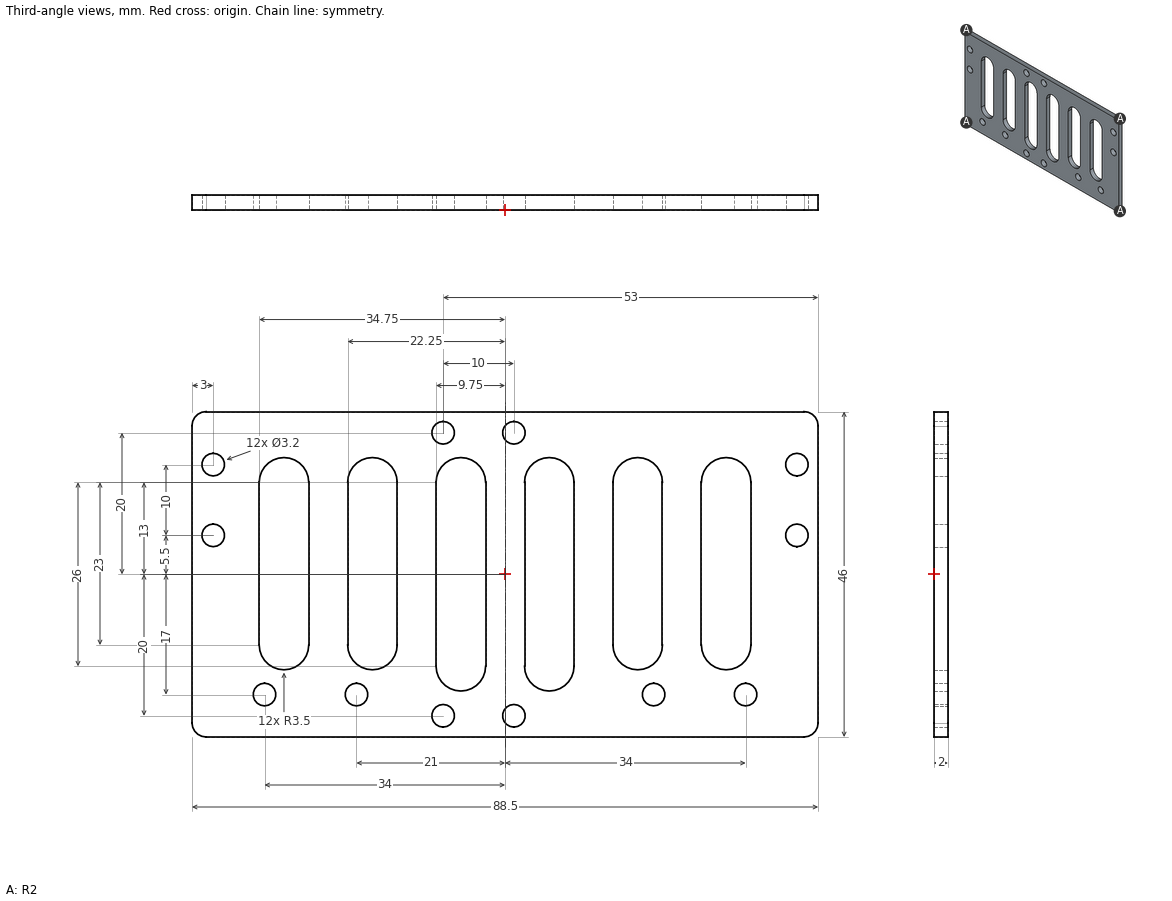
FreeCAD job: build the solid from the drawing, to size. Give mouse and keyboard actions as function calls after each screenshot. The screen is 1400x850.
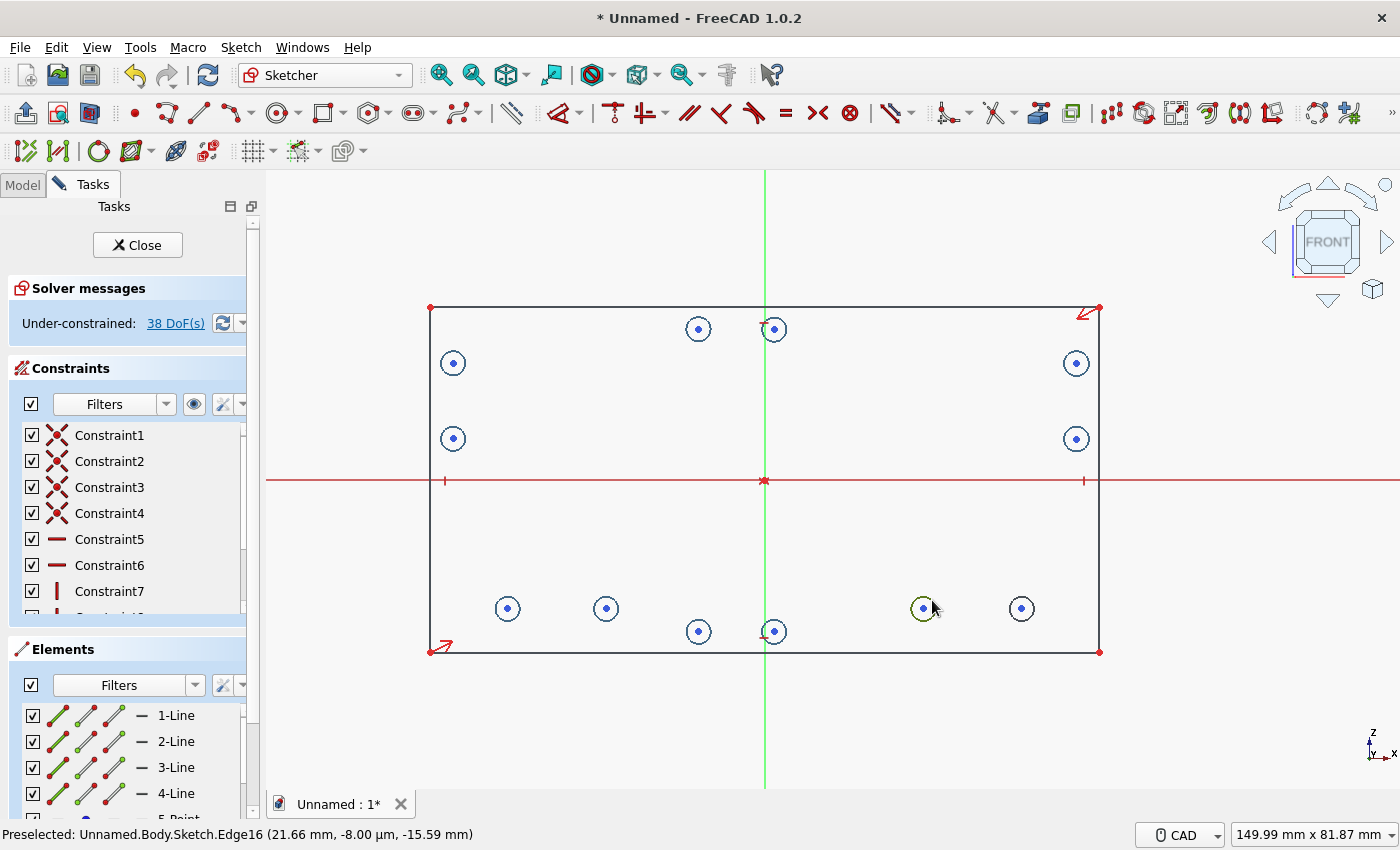
click(1030, 600)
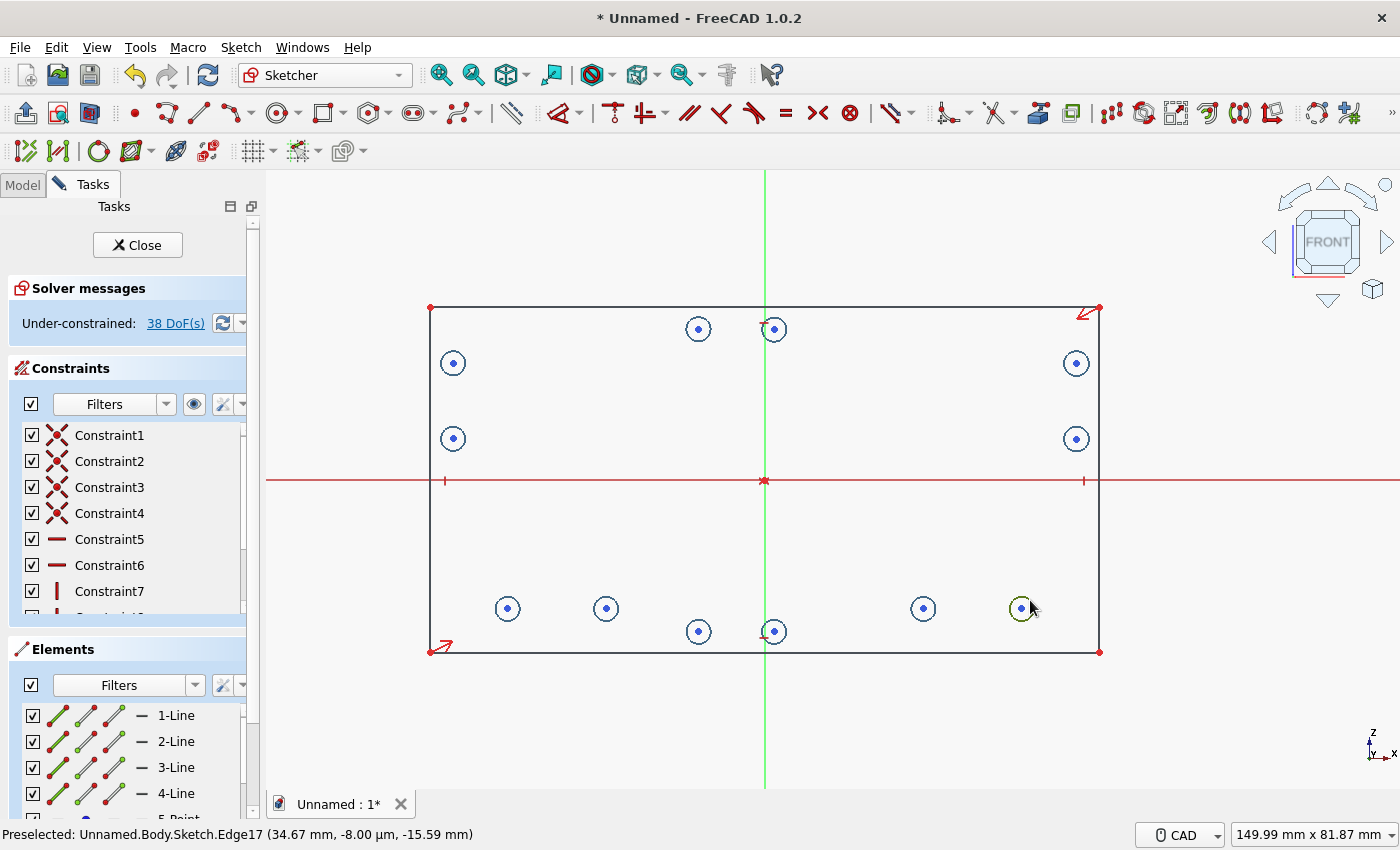
click(786, 114)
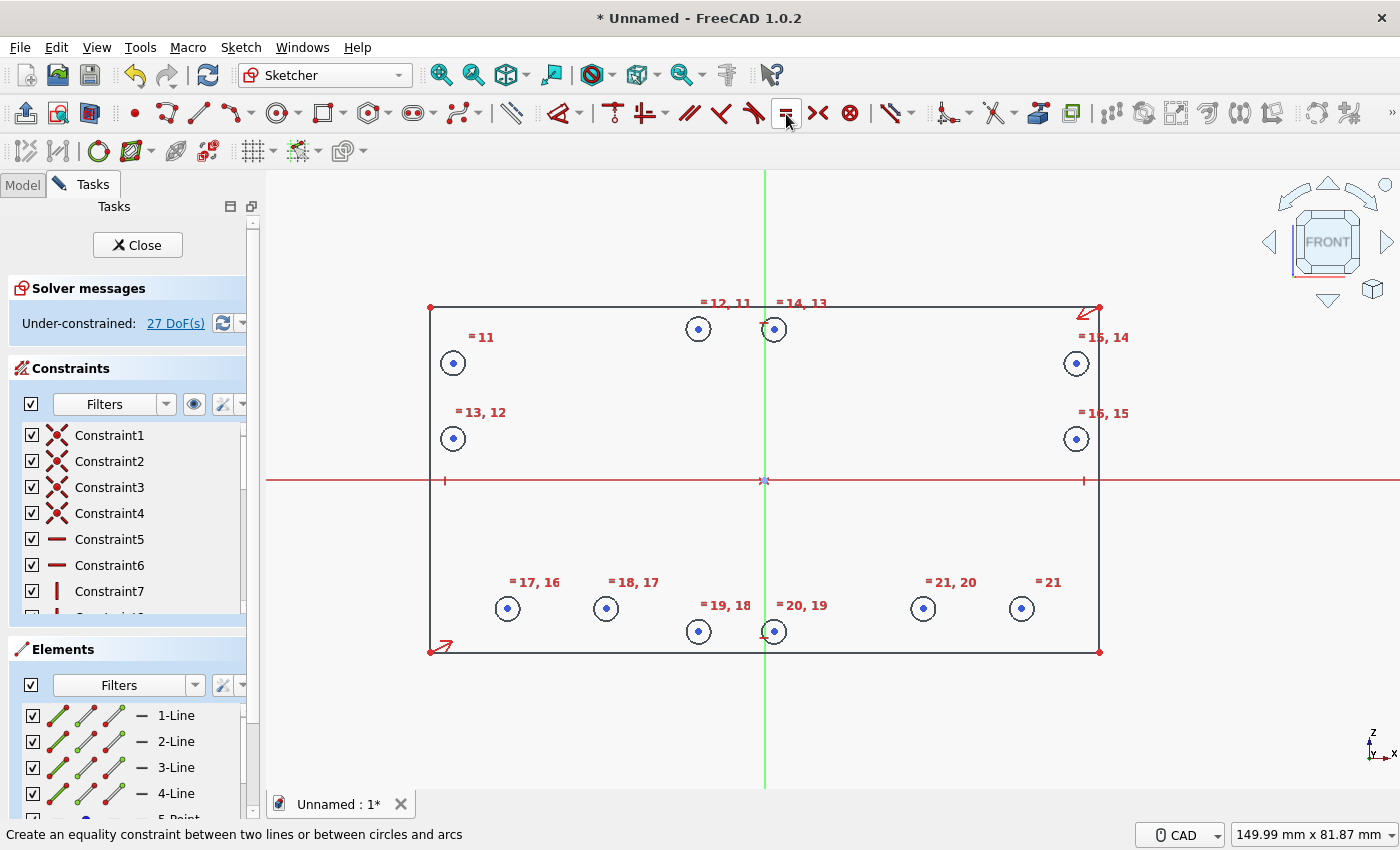
click(453, 363)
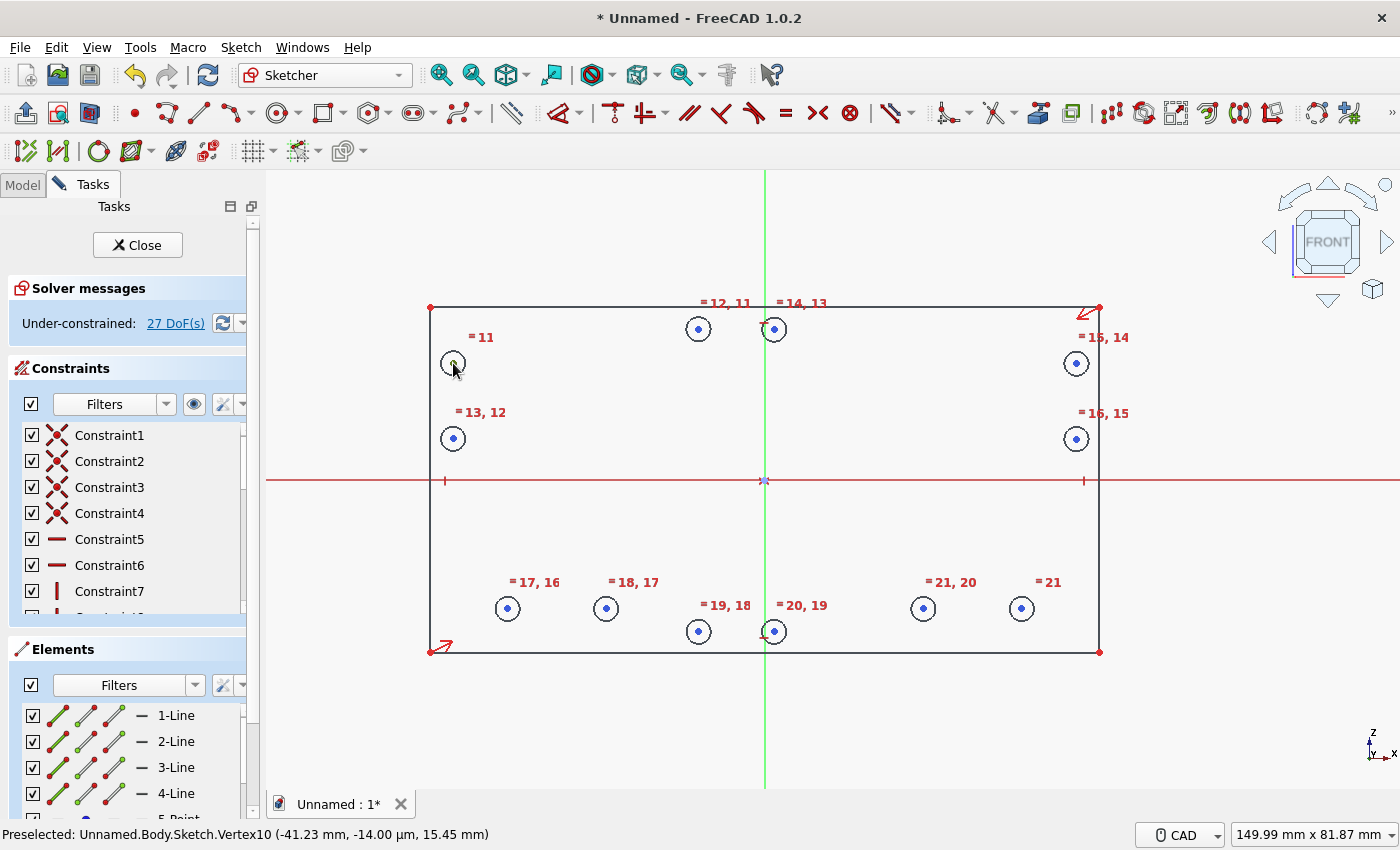
click(453, 439)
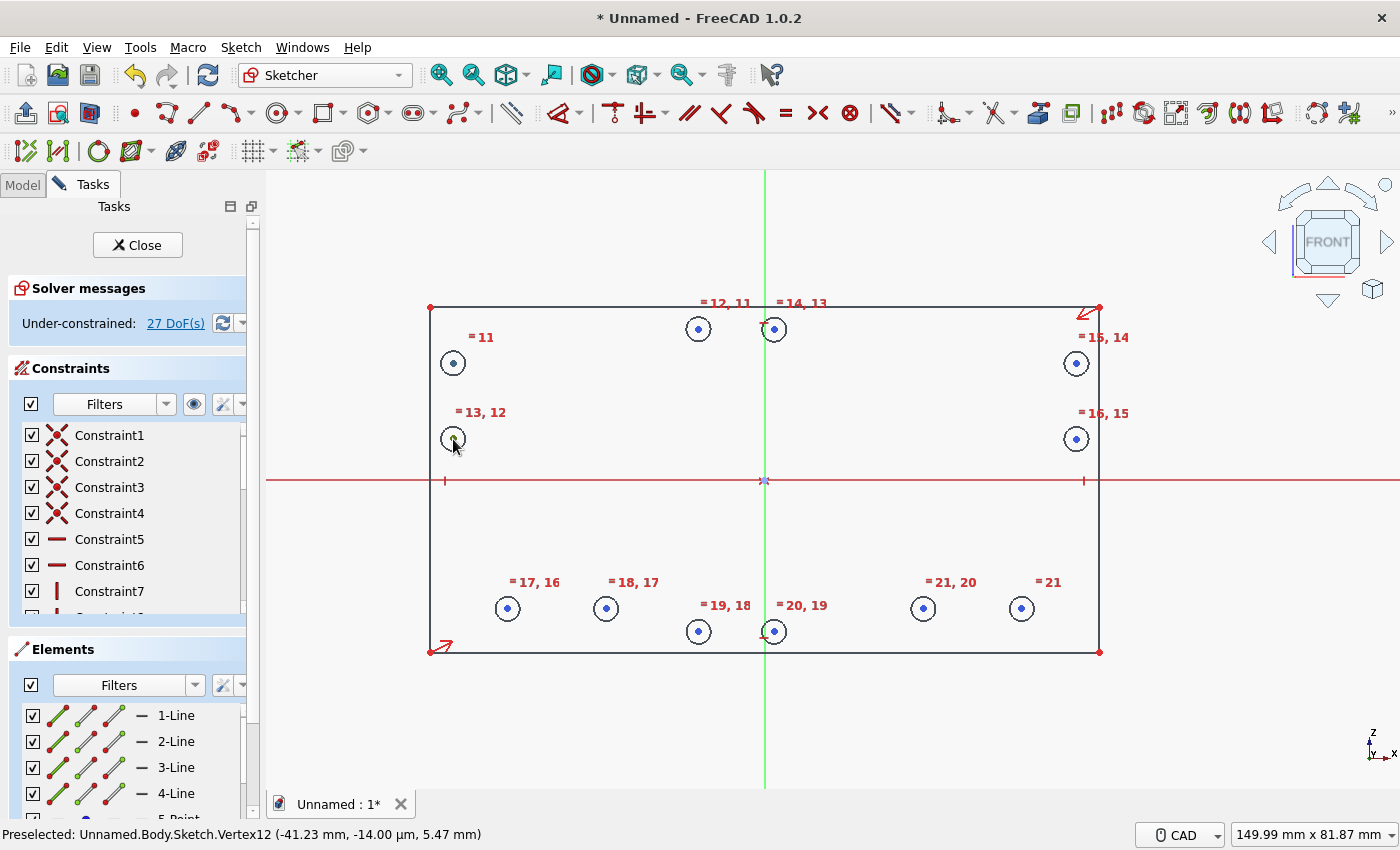
click(668, 114)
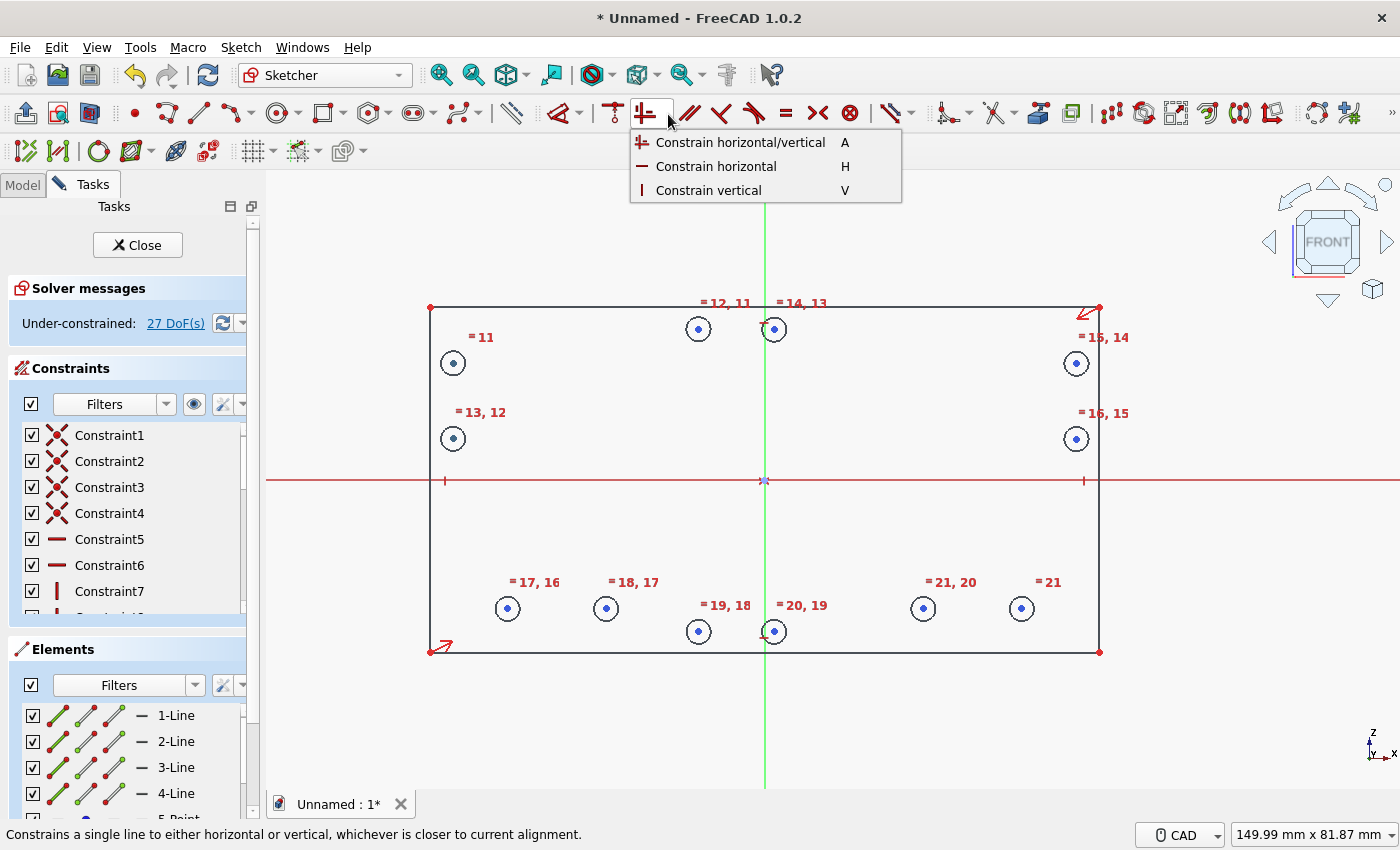
click(766, 190)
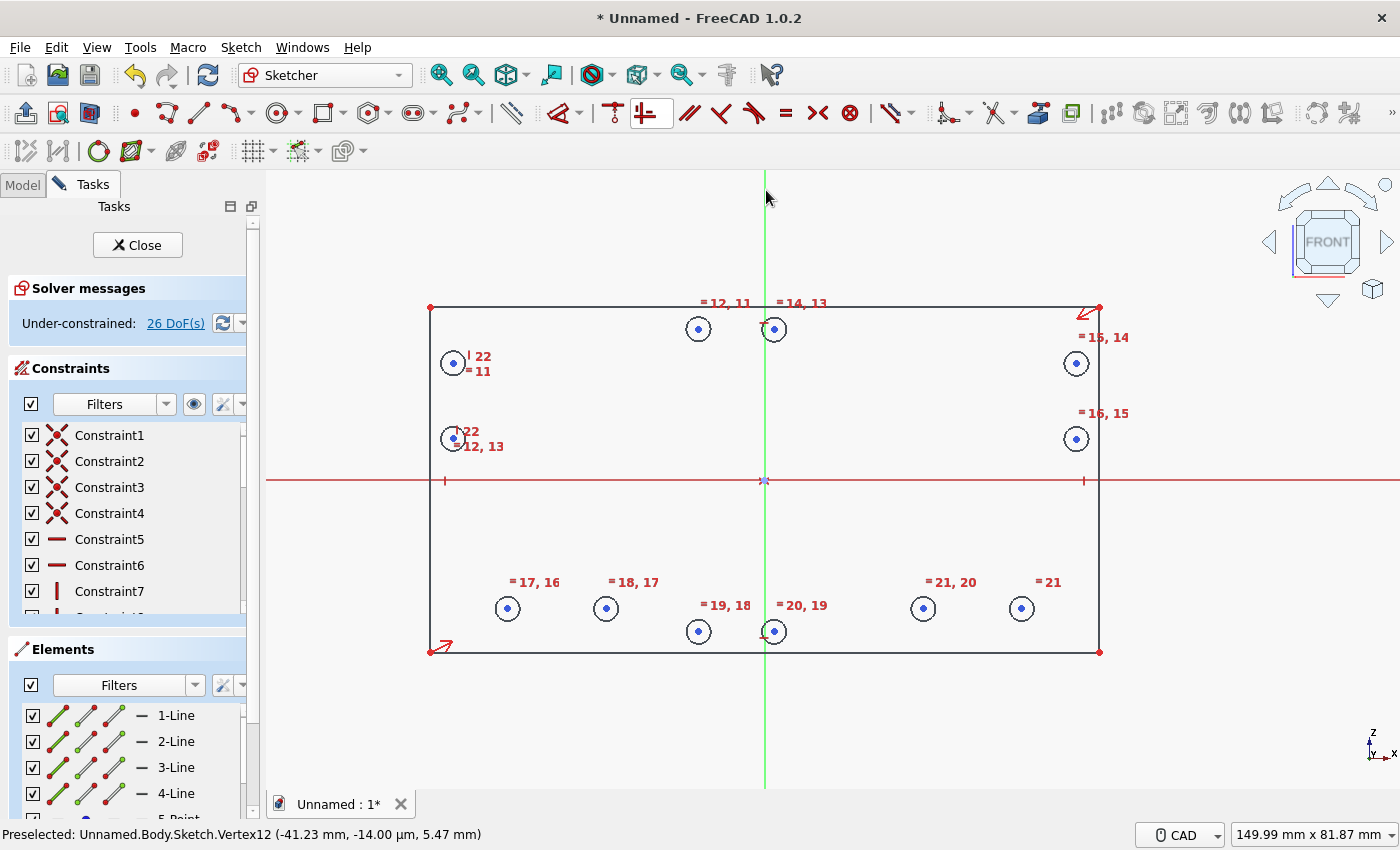
click(698, 329)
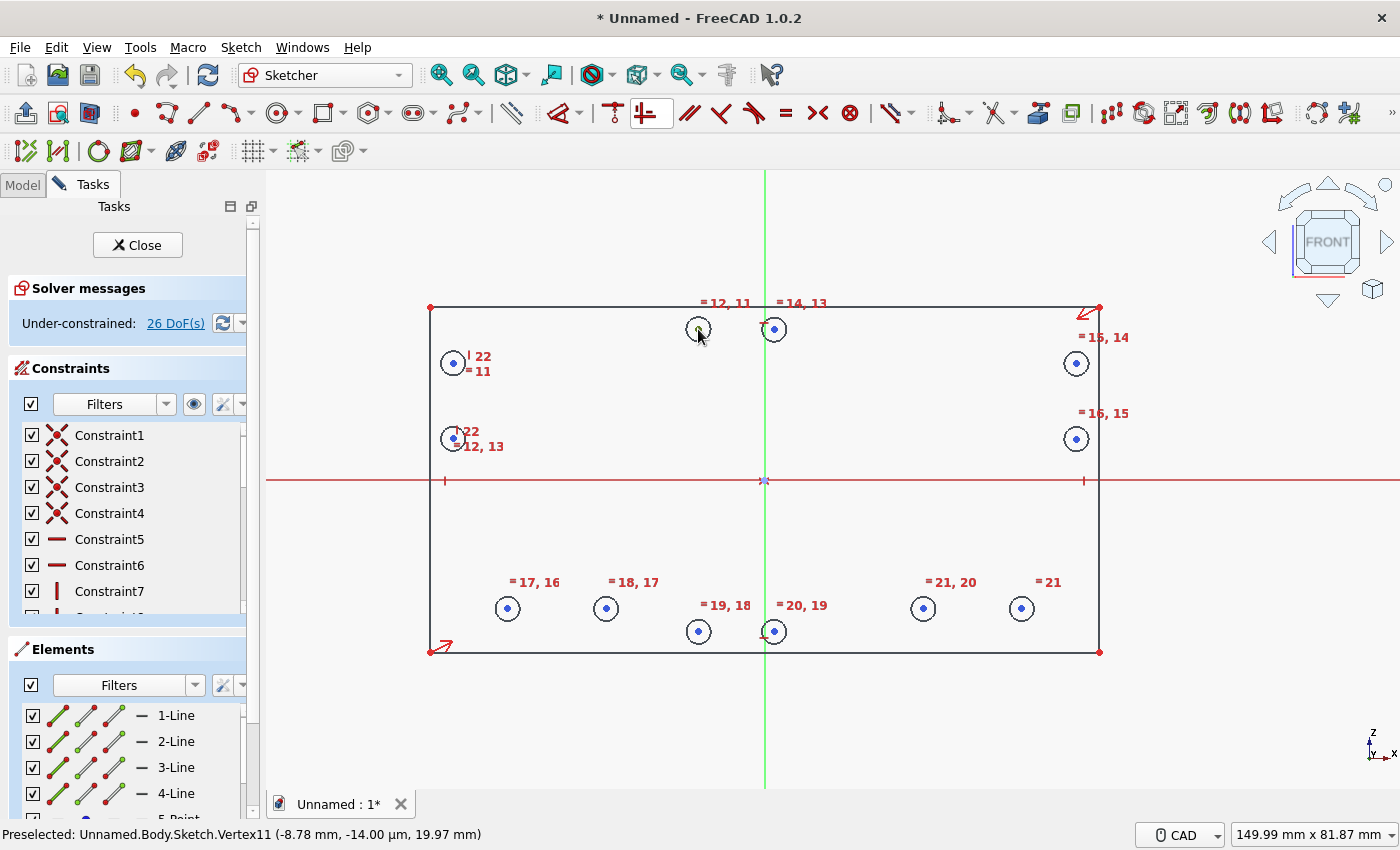
click(774, 330)